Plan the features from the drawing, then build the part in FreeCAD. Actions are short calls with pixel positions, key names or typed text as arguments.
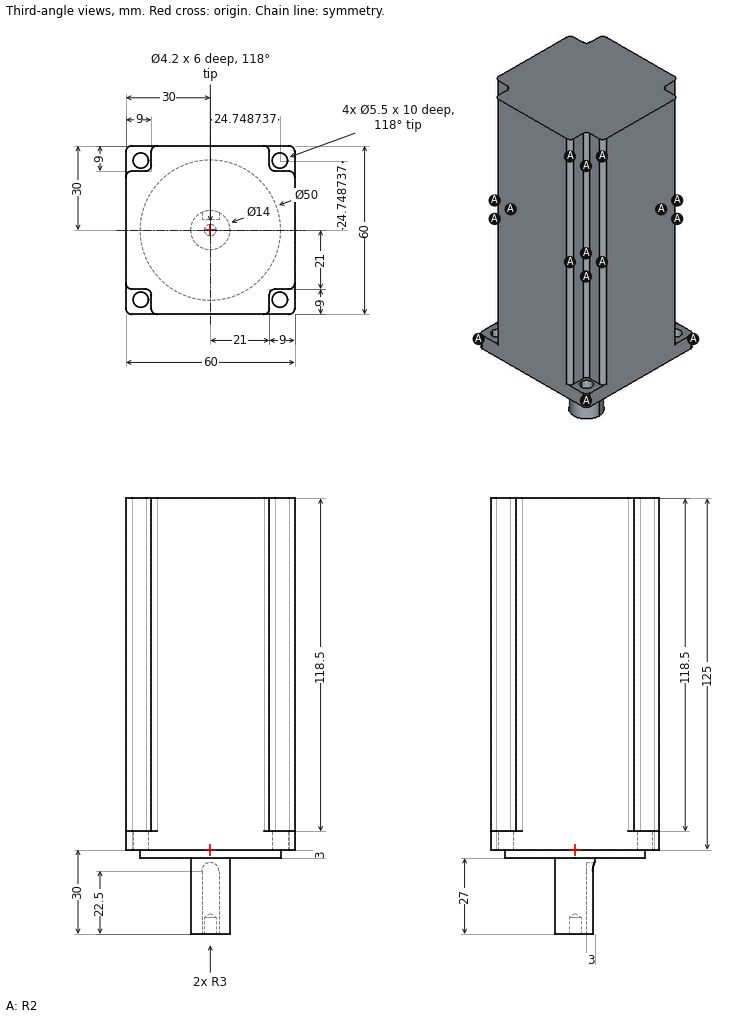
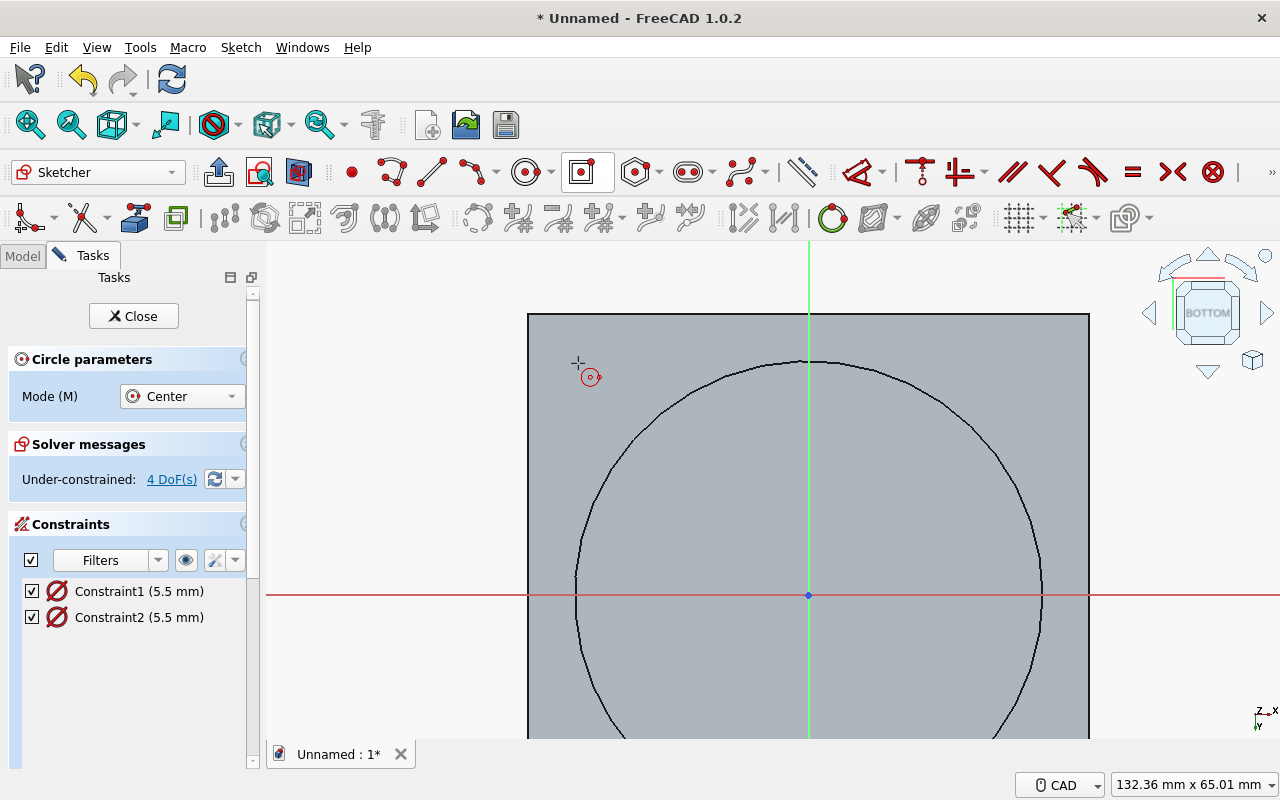
click(577, 364)
move(595, 345)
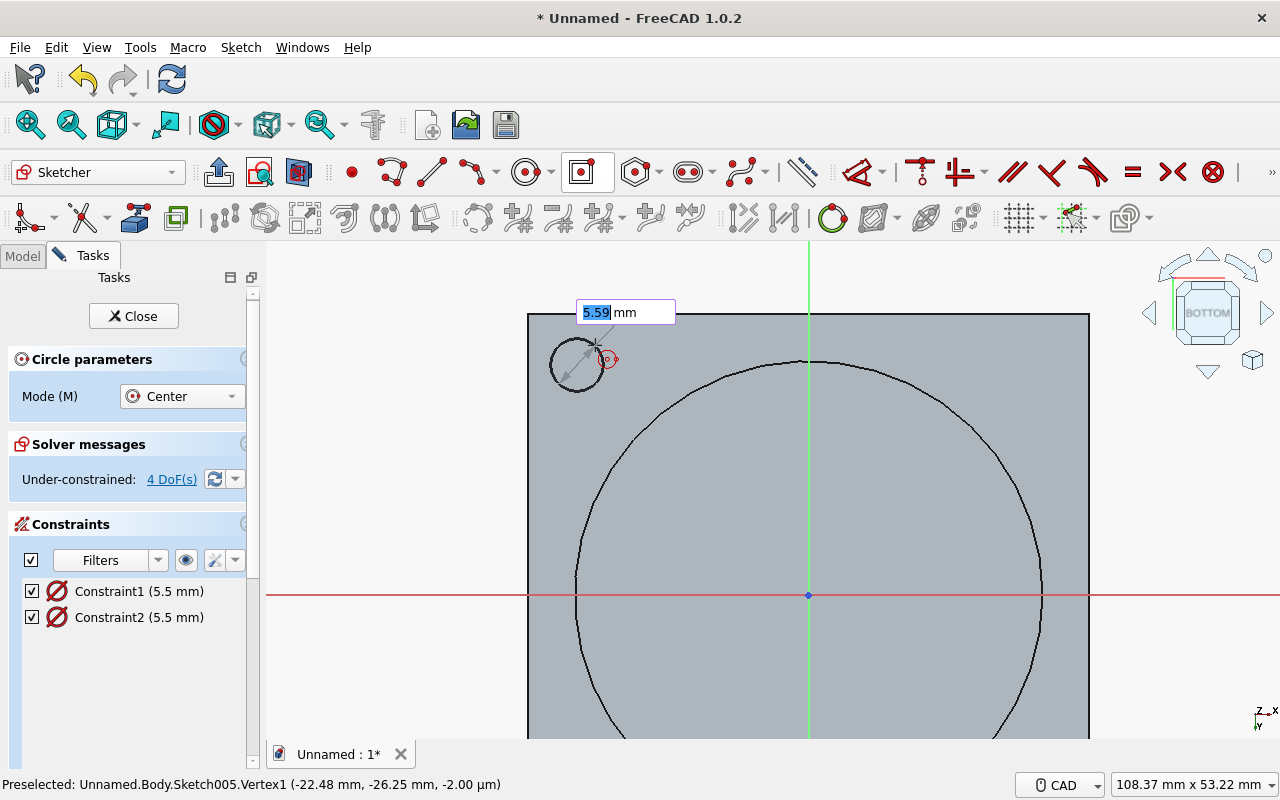
text(5.5)
key(Return)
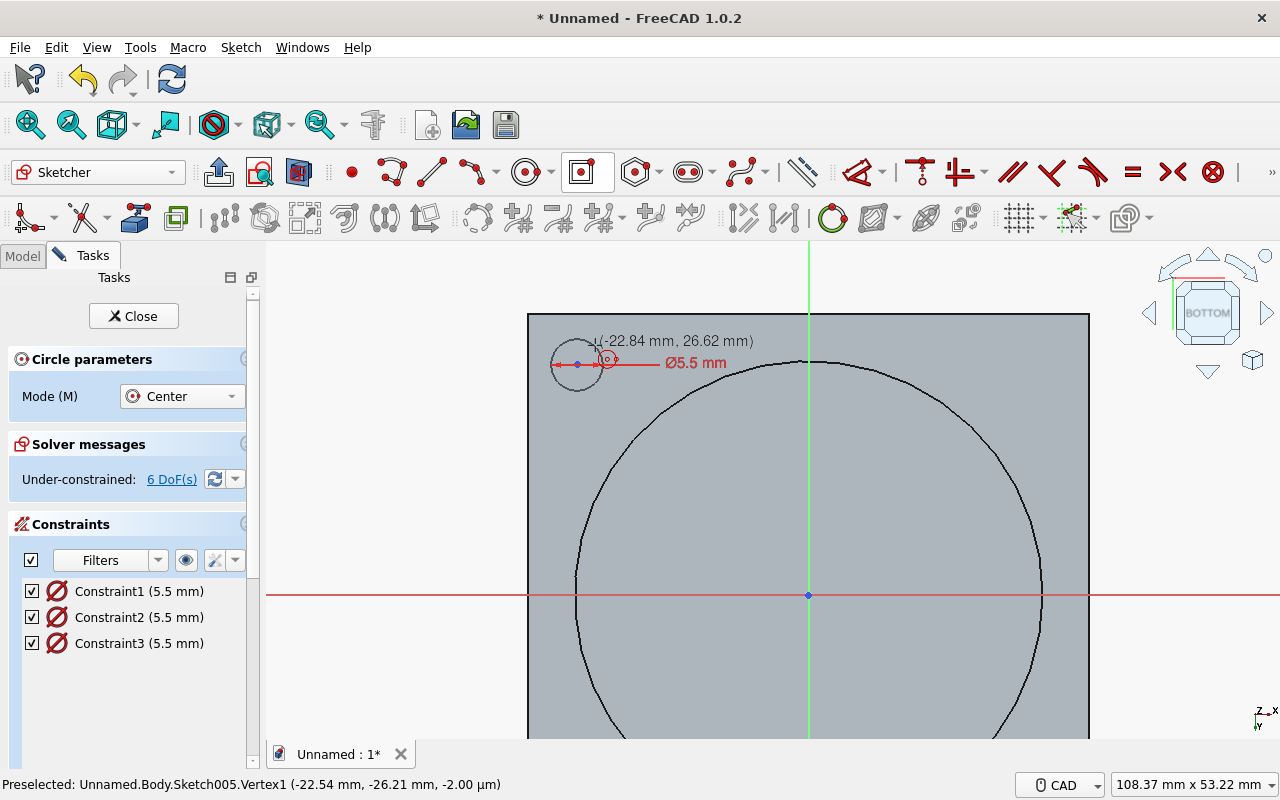
click(1040, 364)
move(1058, 345)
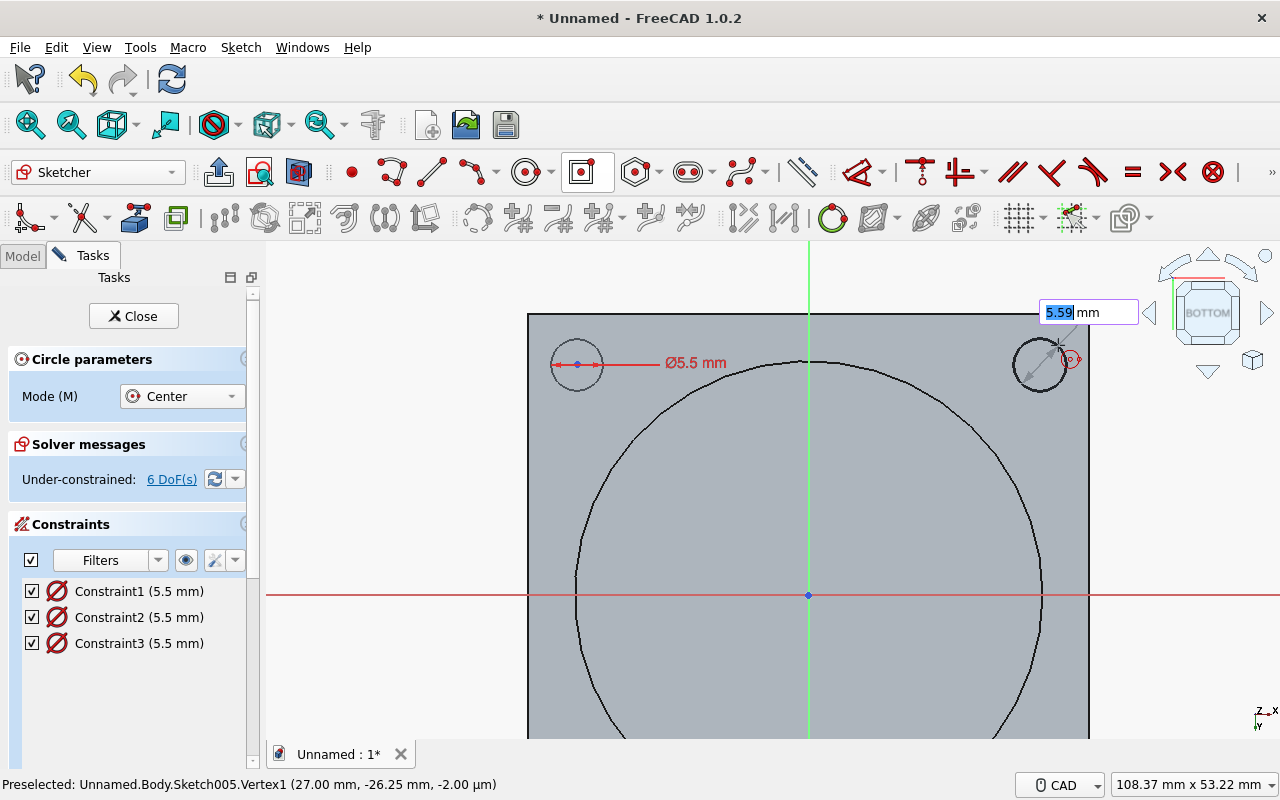
text(5.5)
key(Return)
key(Escape)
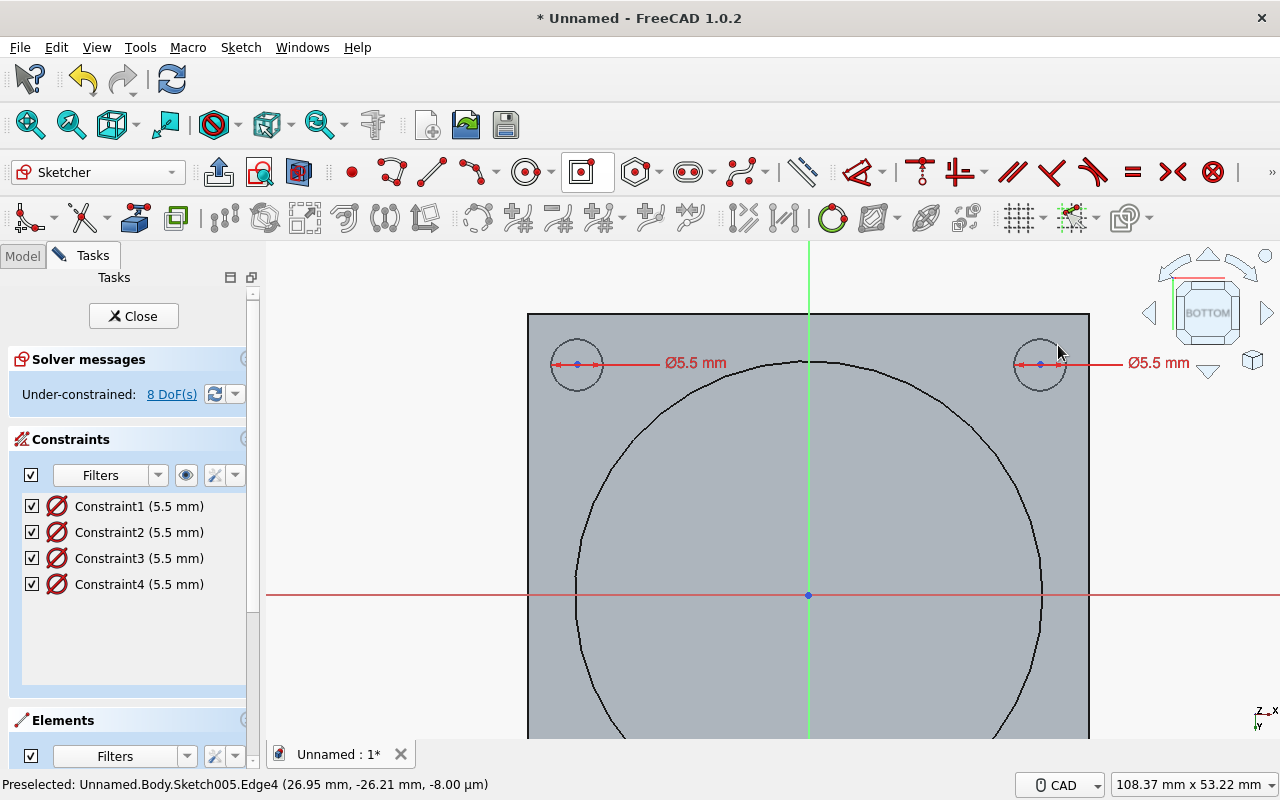
scroll(578, 362, down, 3)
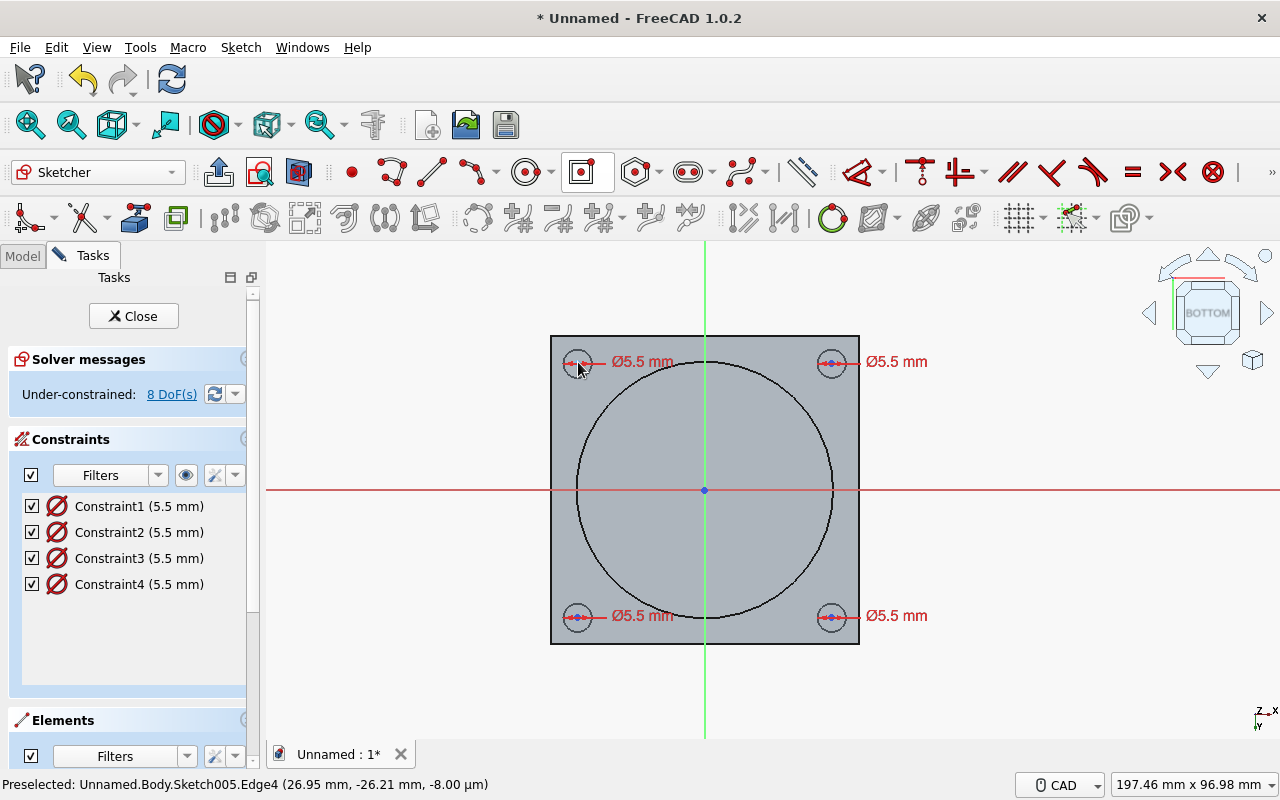
click(832, 618)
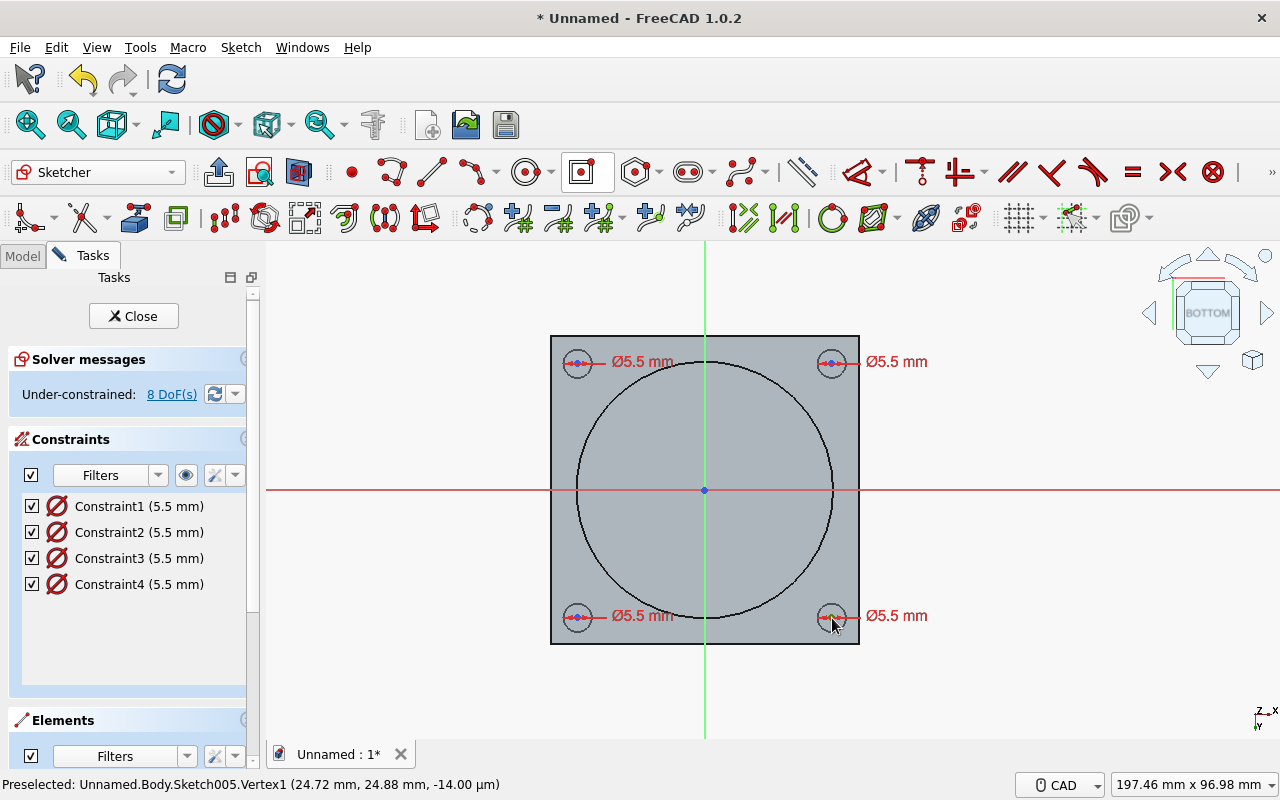
click(578, 618)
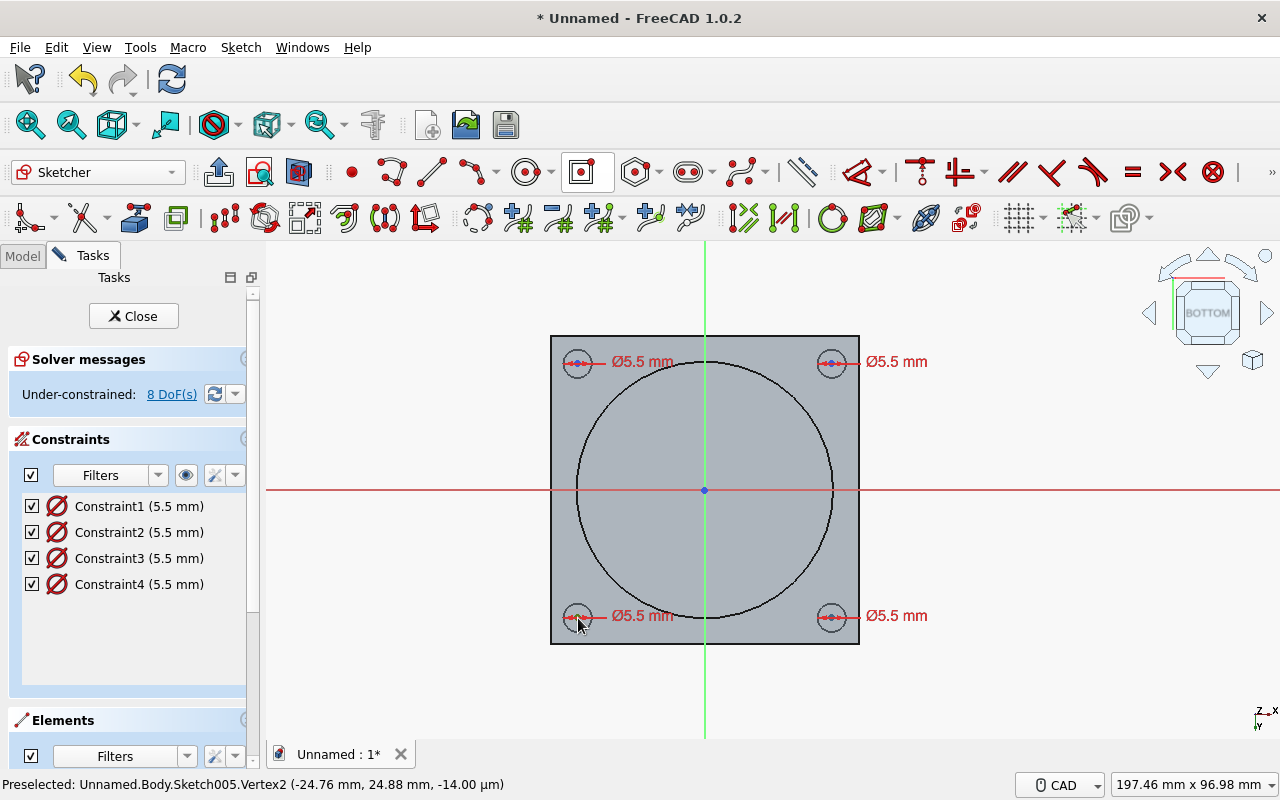
click(705, 679)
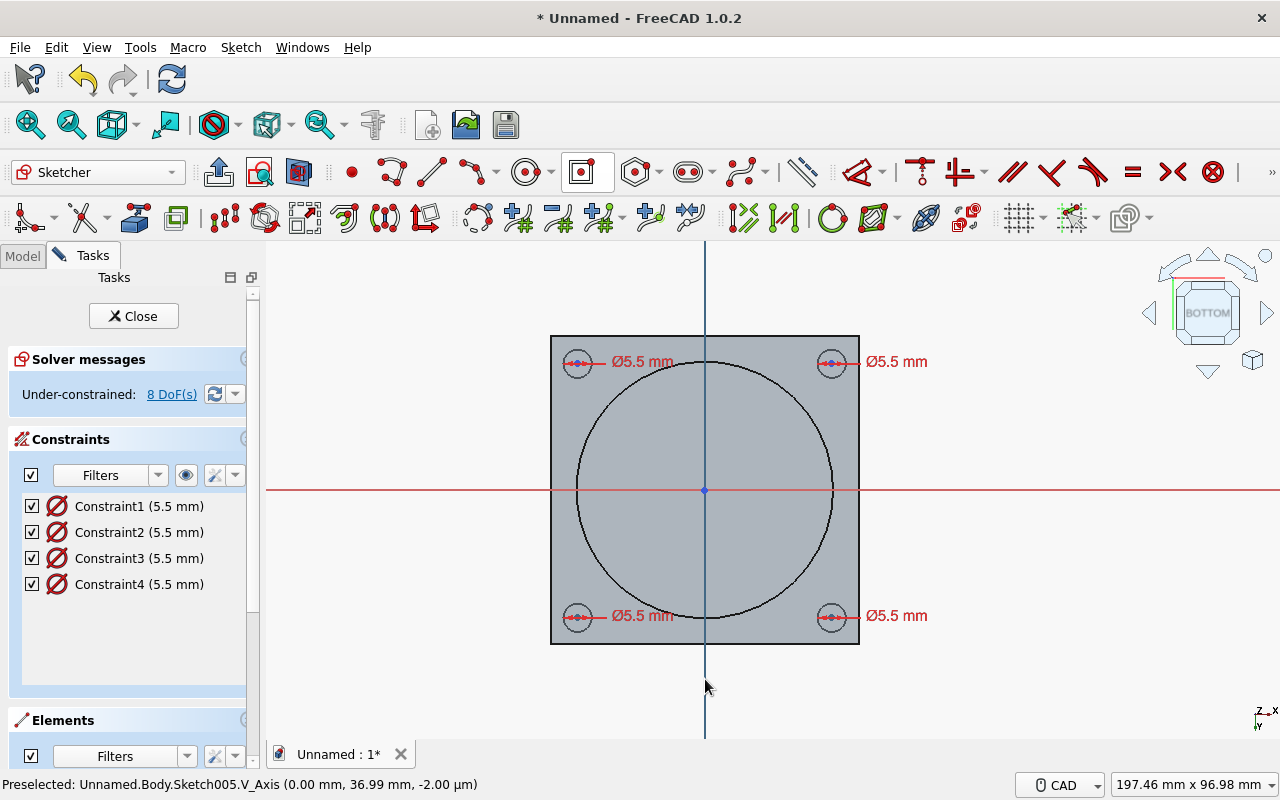
click(1174, 172)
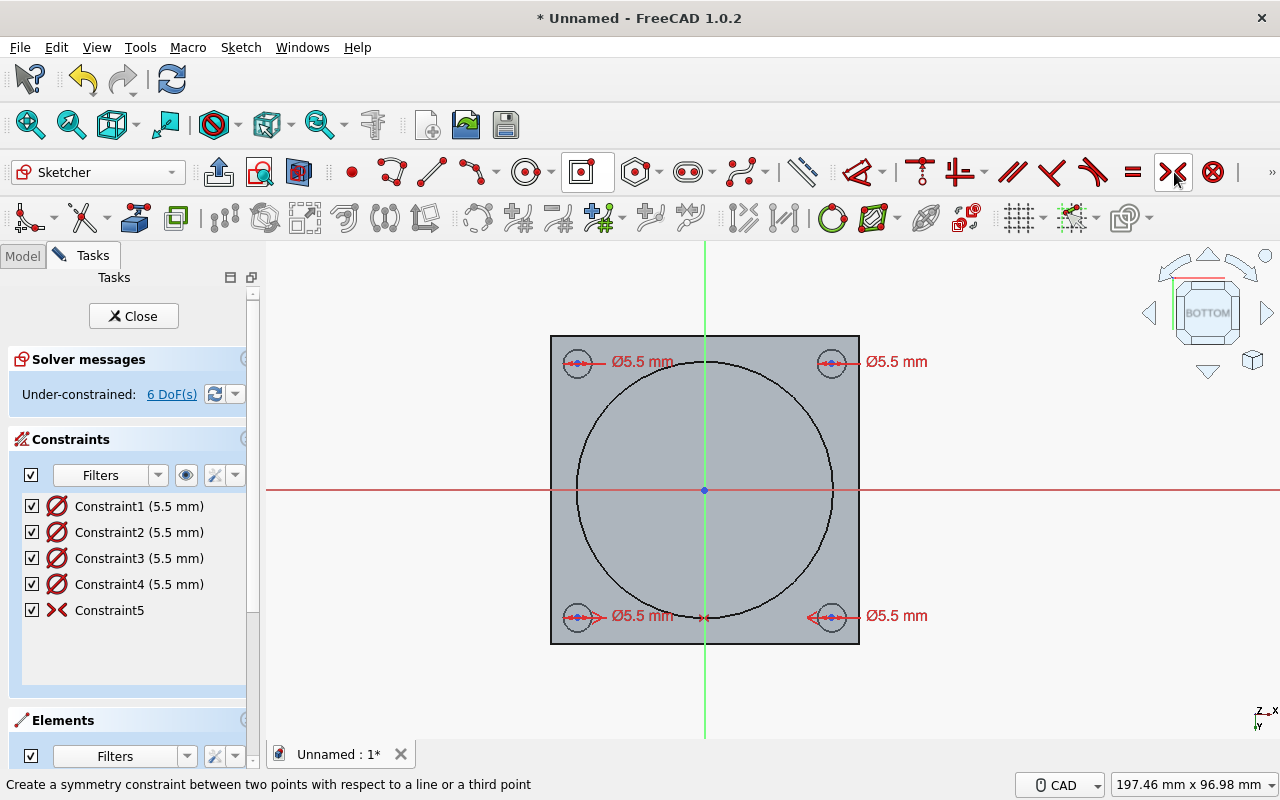
click(578, 618)